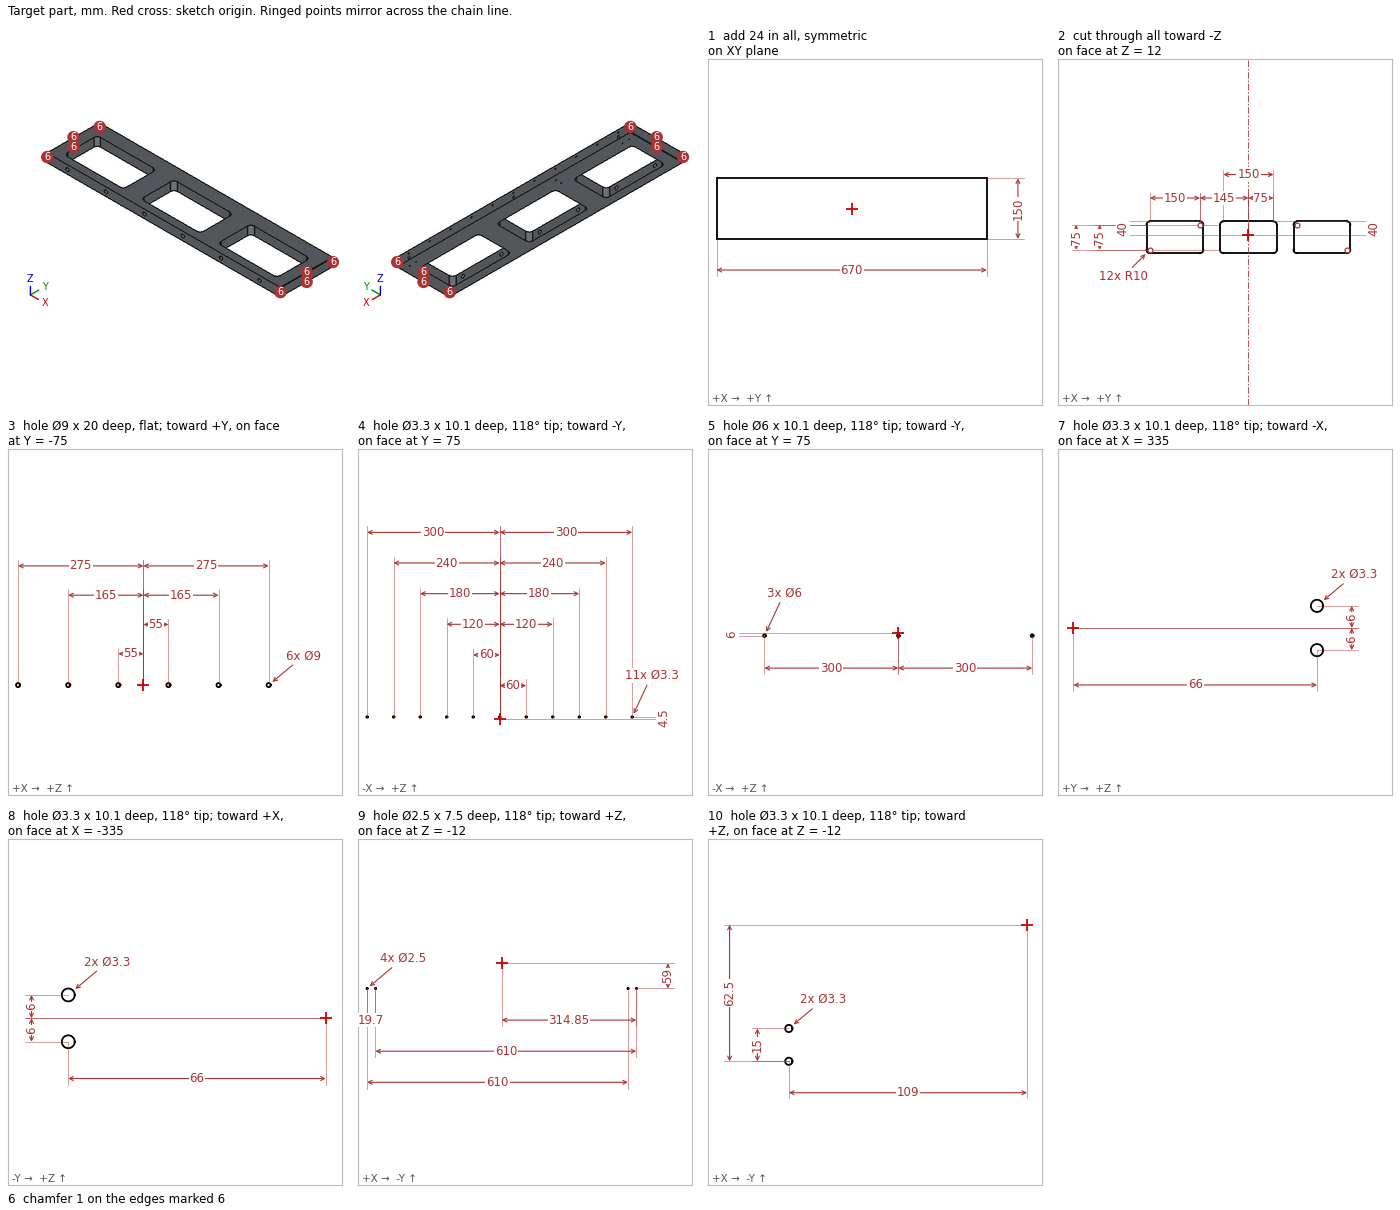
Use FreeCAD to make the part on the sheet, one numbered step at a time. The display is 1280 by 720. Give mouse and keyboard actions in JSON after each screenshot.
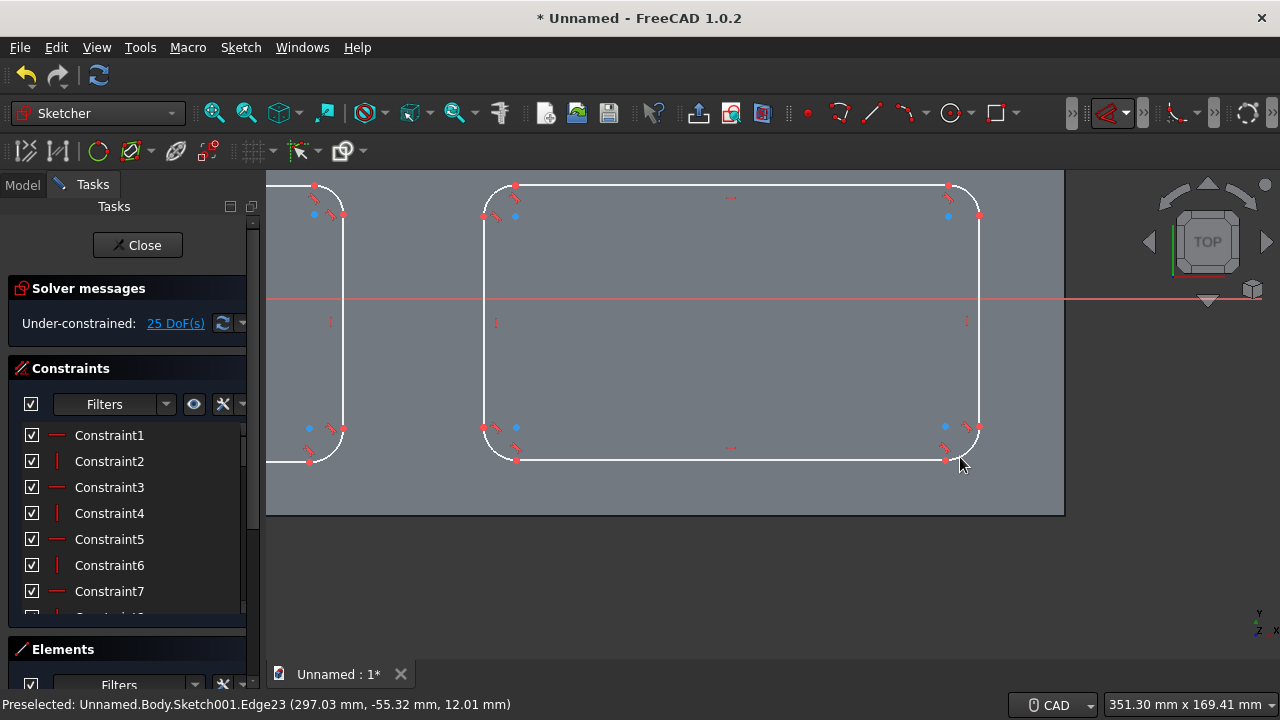
{"action": "scroll", "coordinate": [966, 455], "scroll_direction": "down", "scroll_amount": 6}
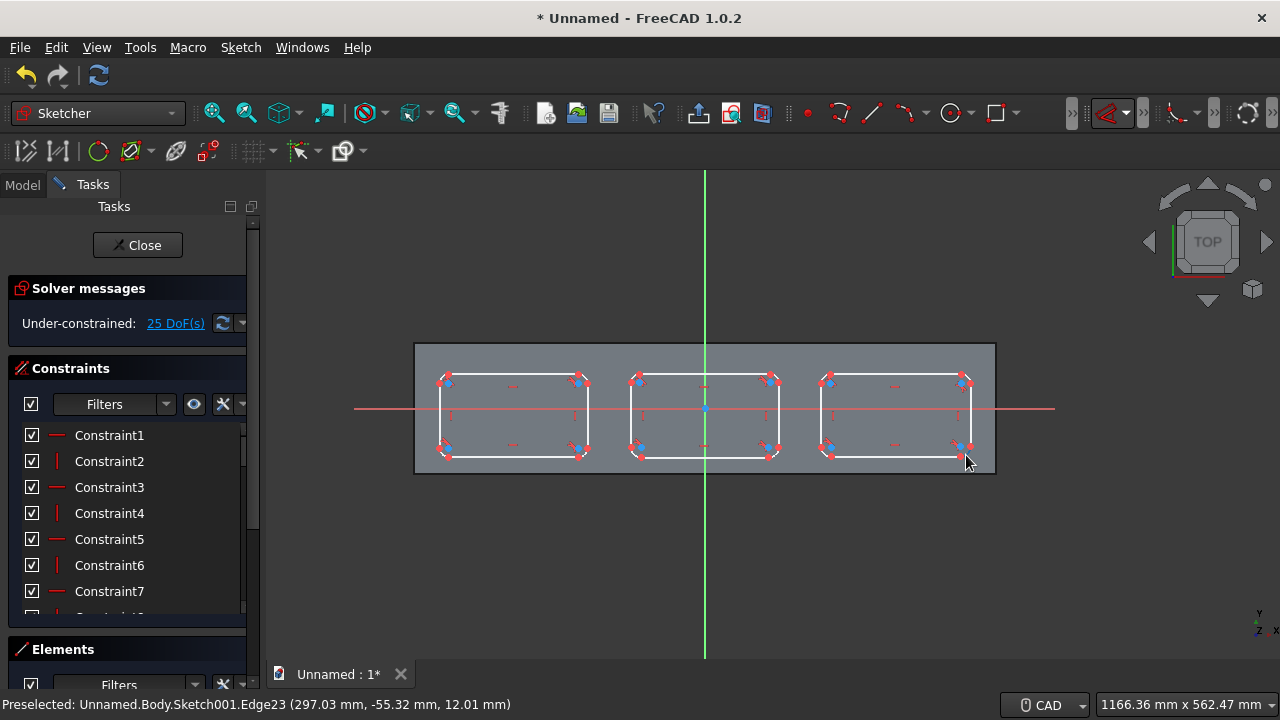
{"action": "left_click", "coordinate": [971, 428]}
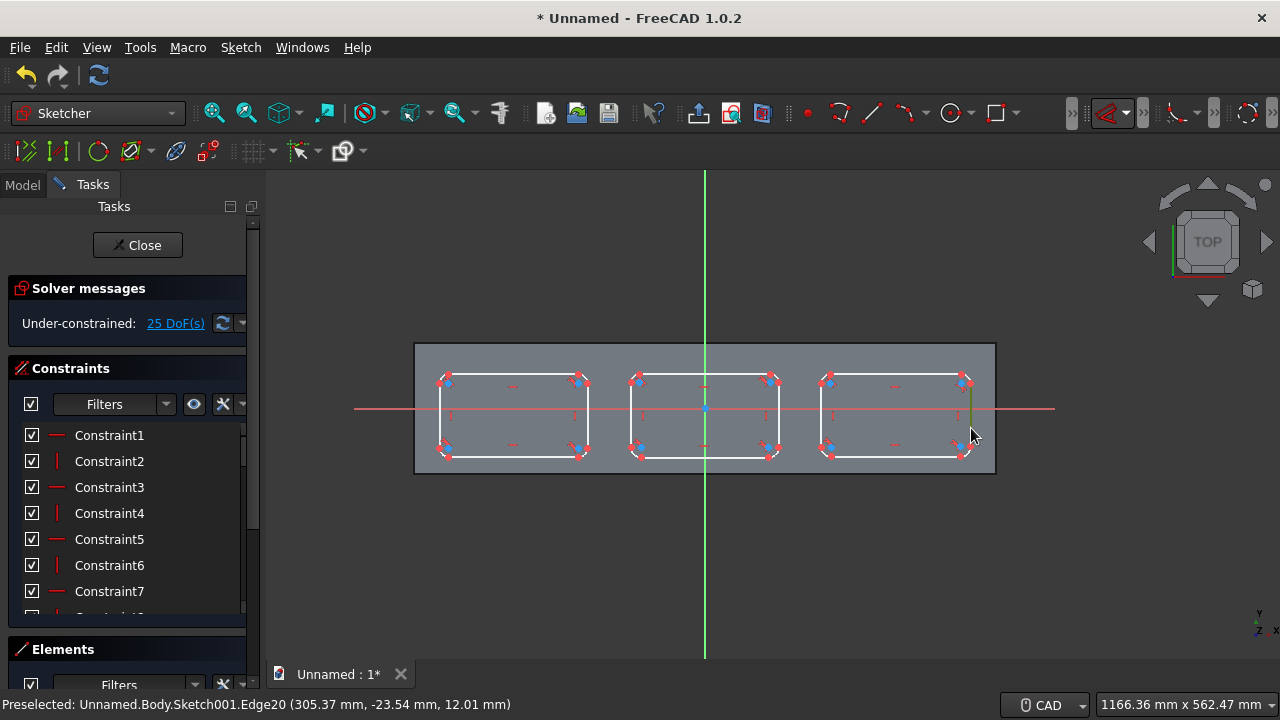
{"action": "scroll", "coordinate": [968, 377], "scroll_direction": "up", "scroll_amount": 4}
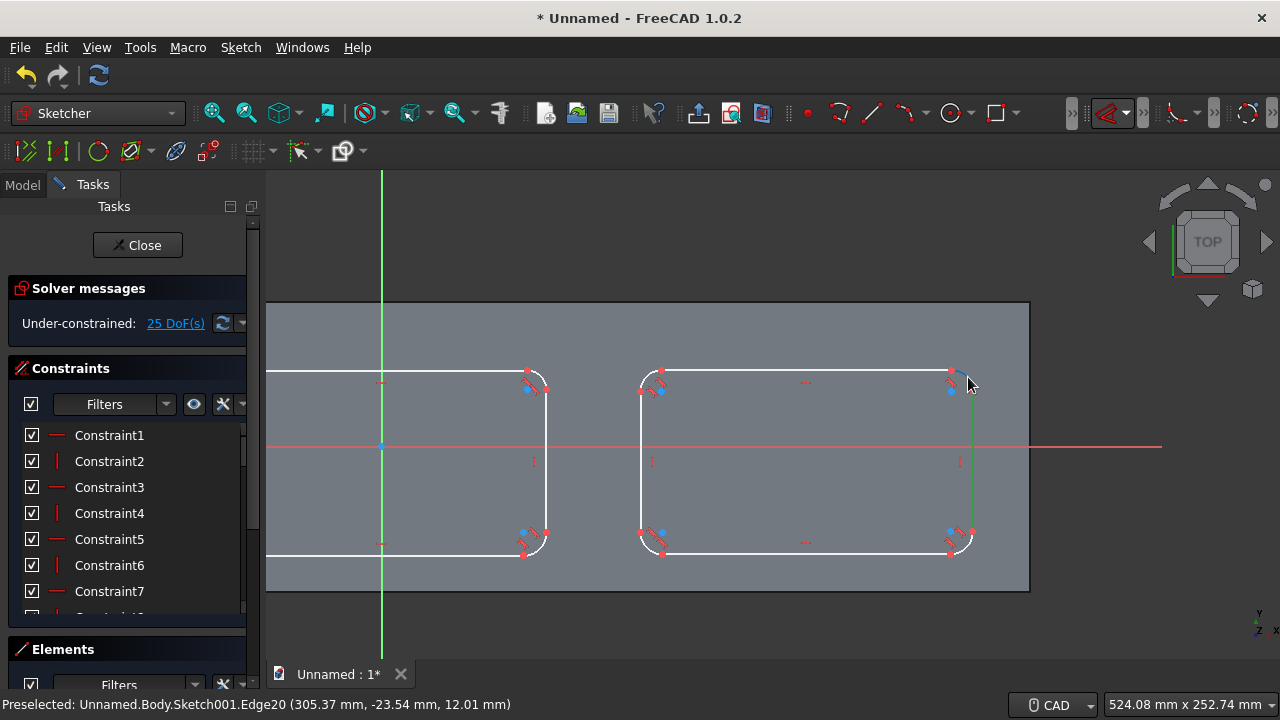
{"action": "left_click", "coordinate": [966, 376]}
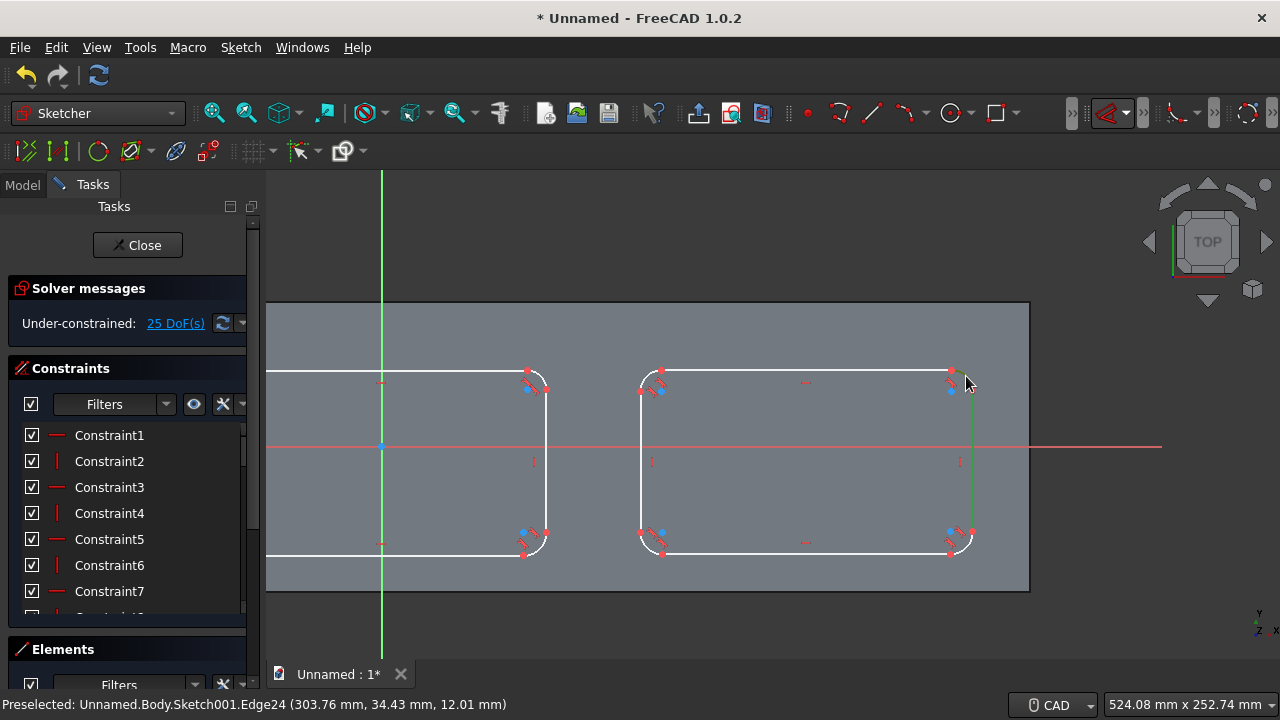
{"action": "key", "text": "t"}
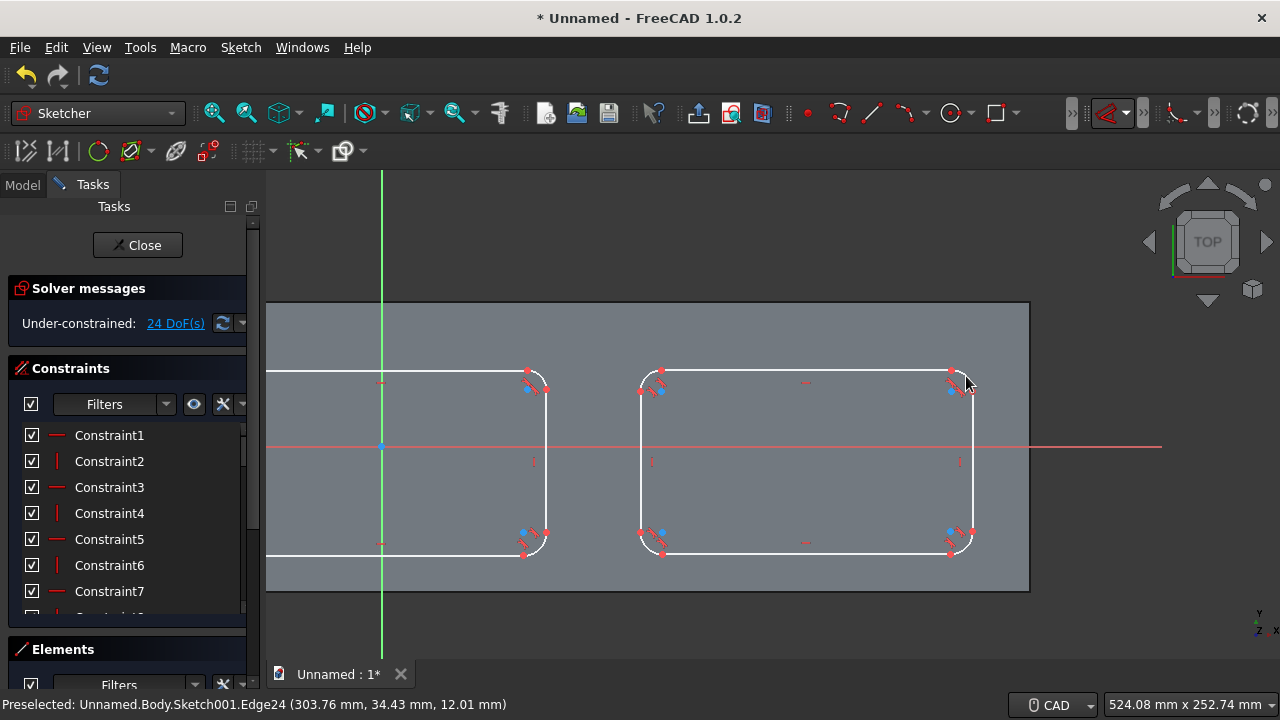
{"action": "scroll", "coordinate": [968, 376], "scroll_direction": "down", "scroll_amount": 4}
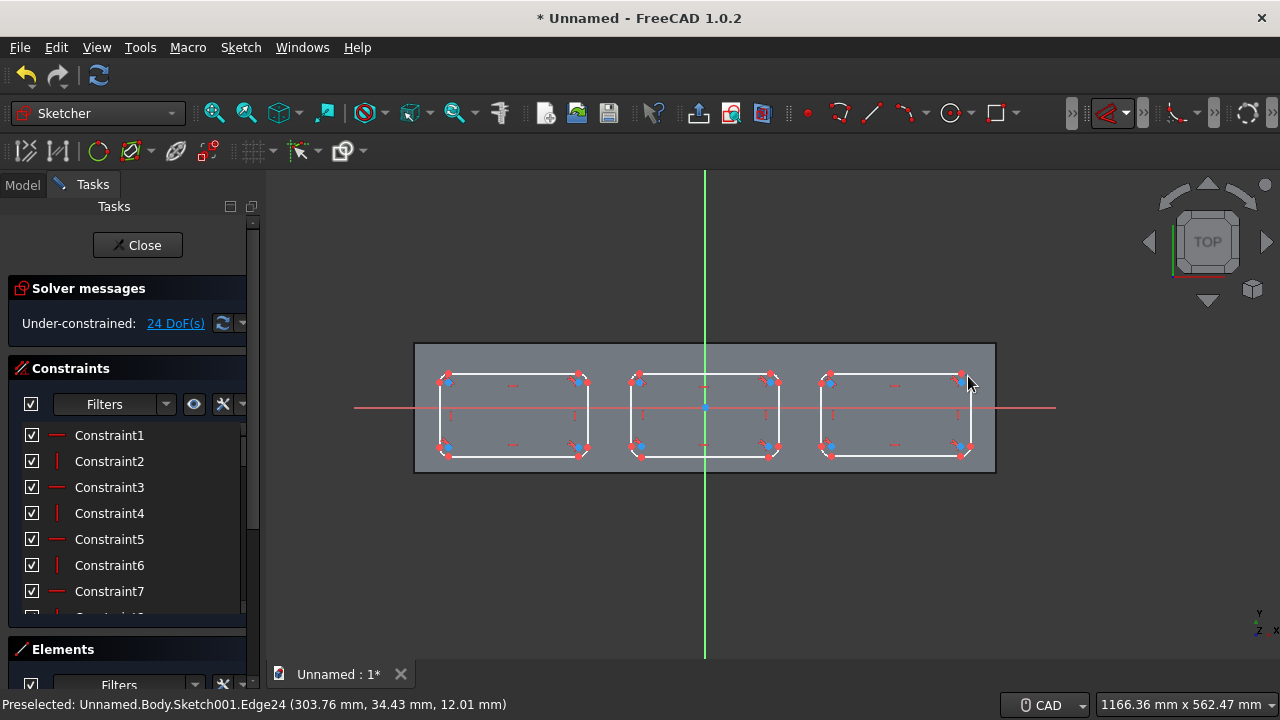
{"action": "scroll", "coordinate": [445, 375], "scroll_direction": "up", "scroll_amount": 6}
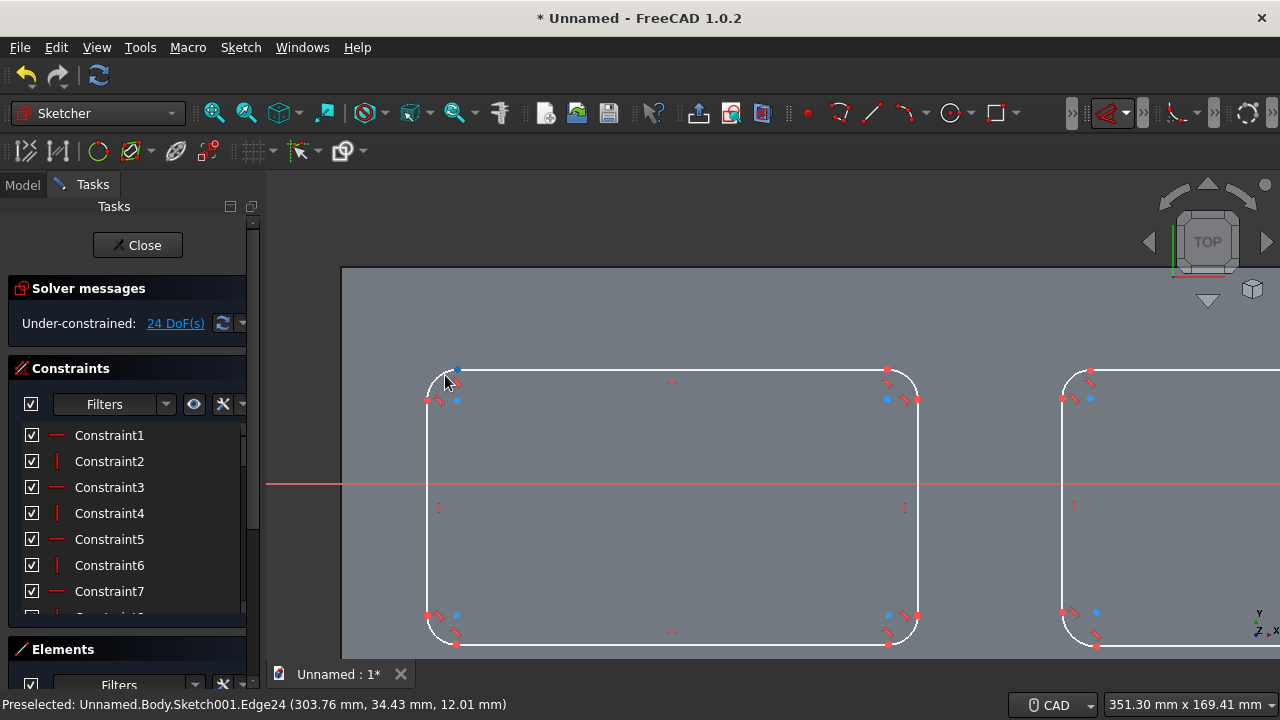
{"action": "left_click", "coordinate": [444, 373]}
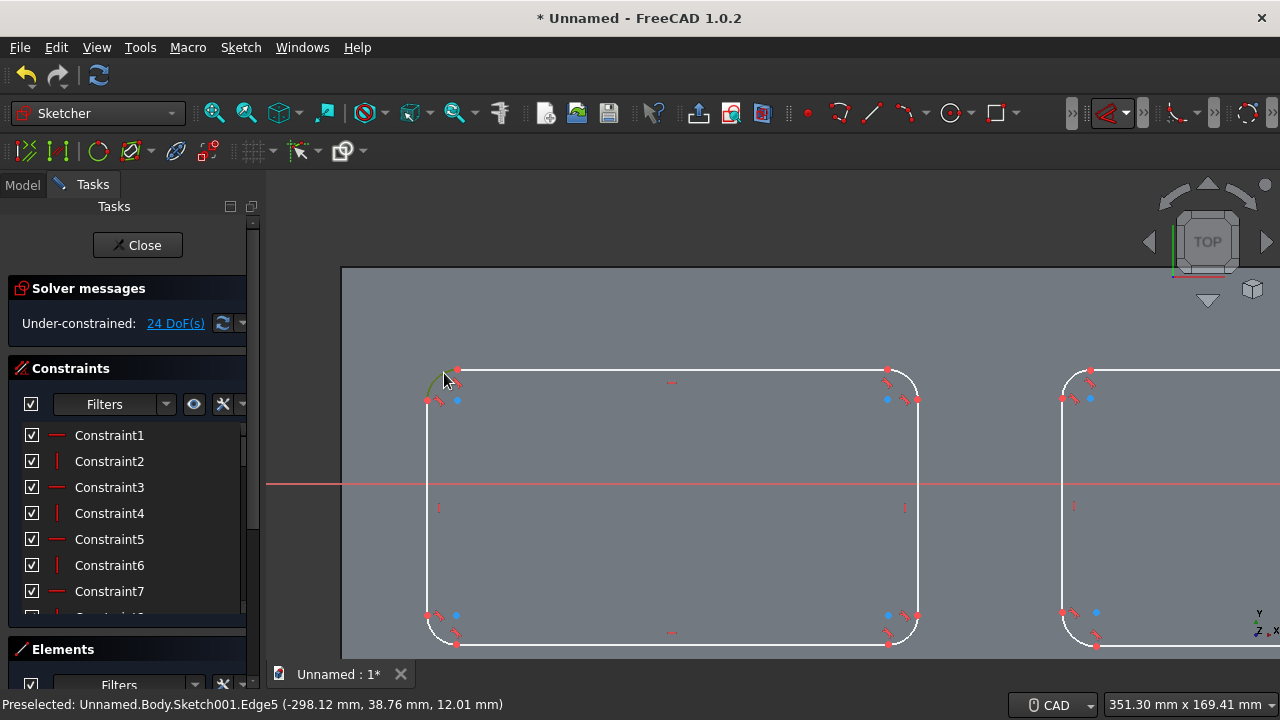
{"action": "left_click", "coordinate": [430, 629]}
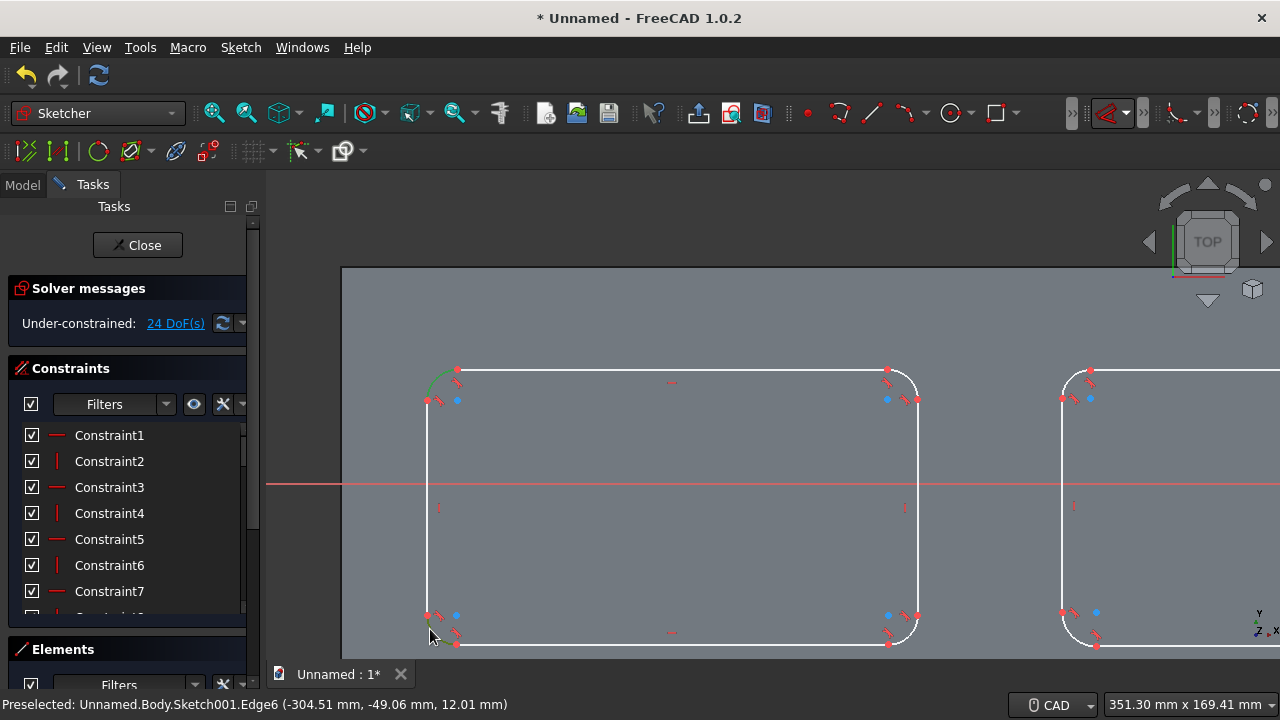
{"action": "left_click", "coordinate": [915, 629]}